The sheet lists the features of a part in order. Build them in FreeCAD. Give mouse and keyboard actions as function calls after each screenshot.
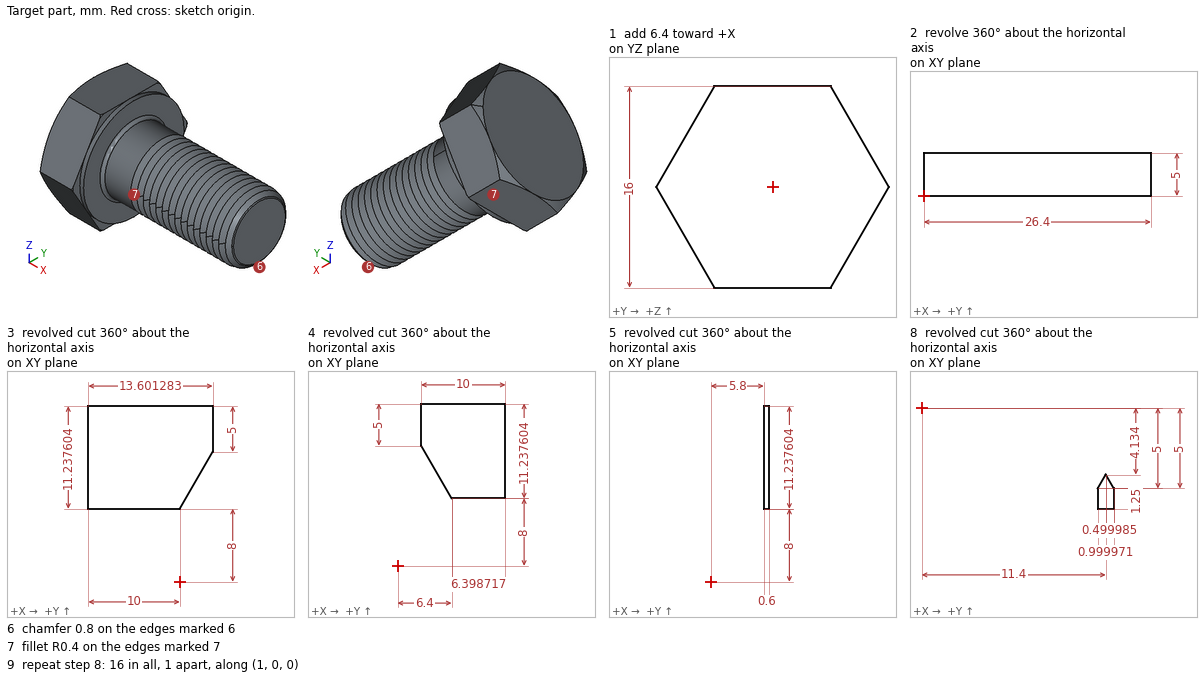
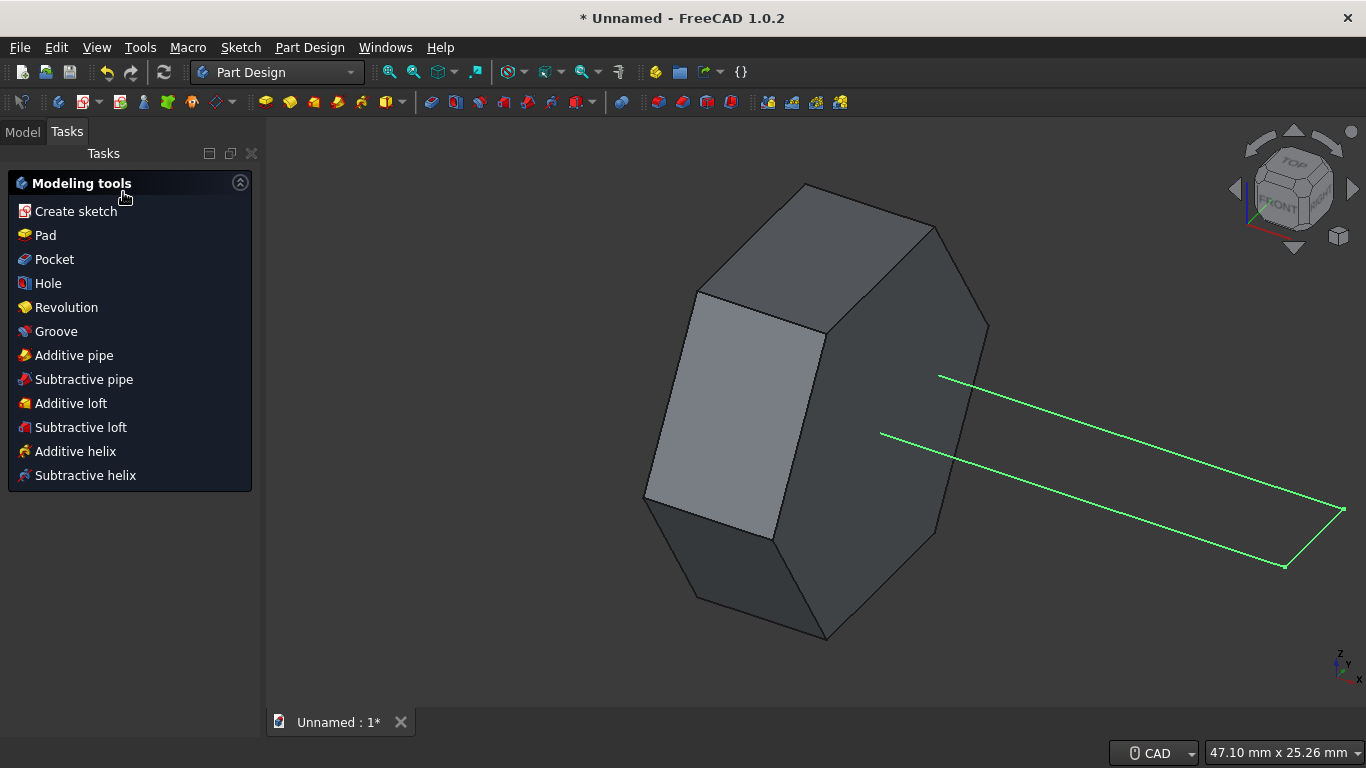
click(290, 102)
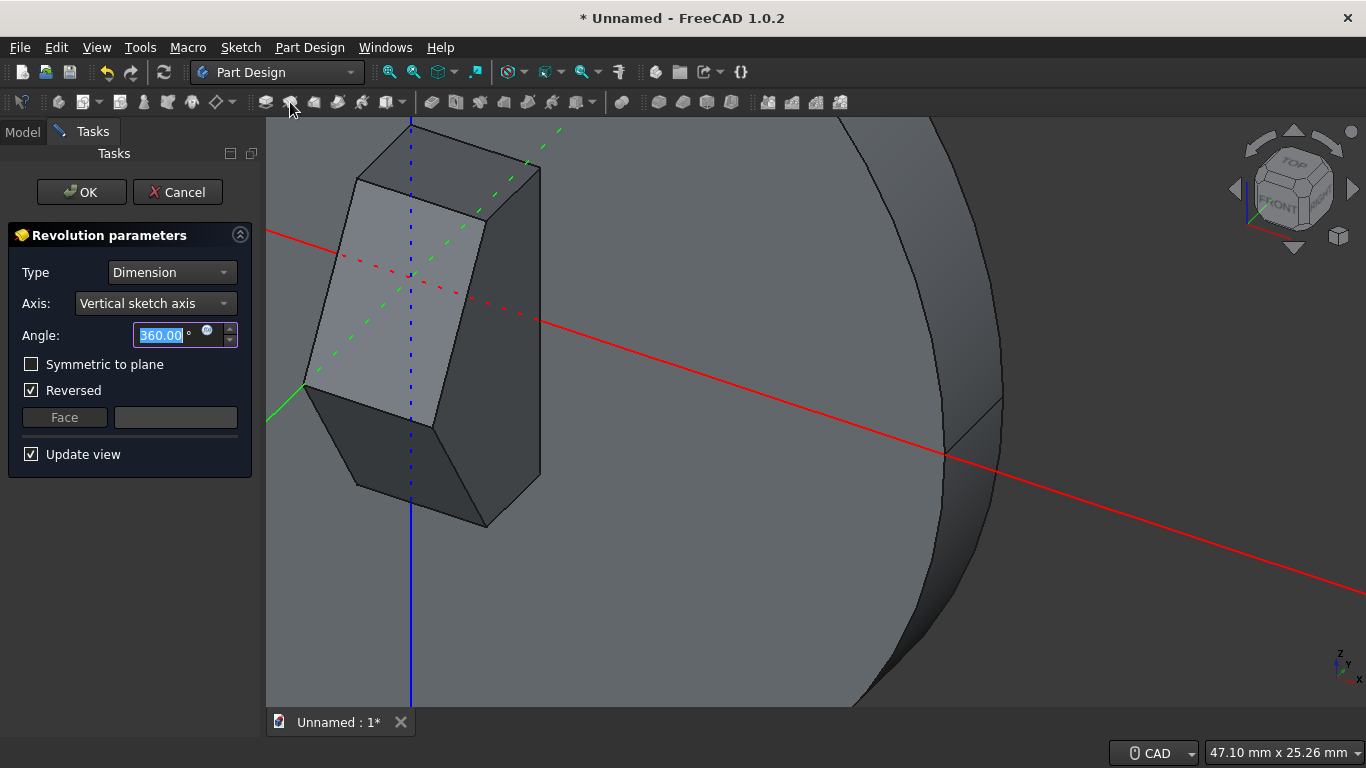
click(156, 304)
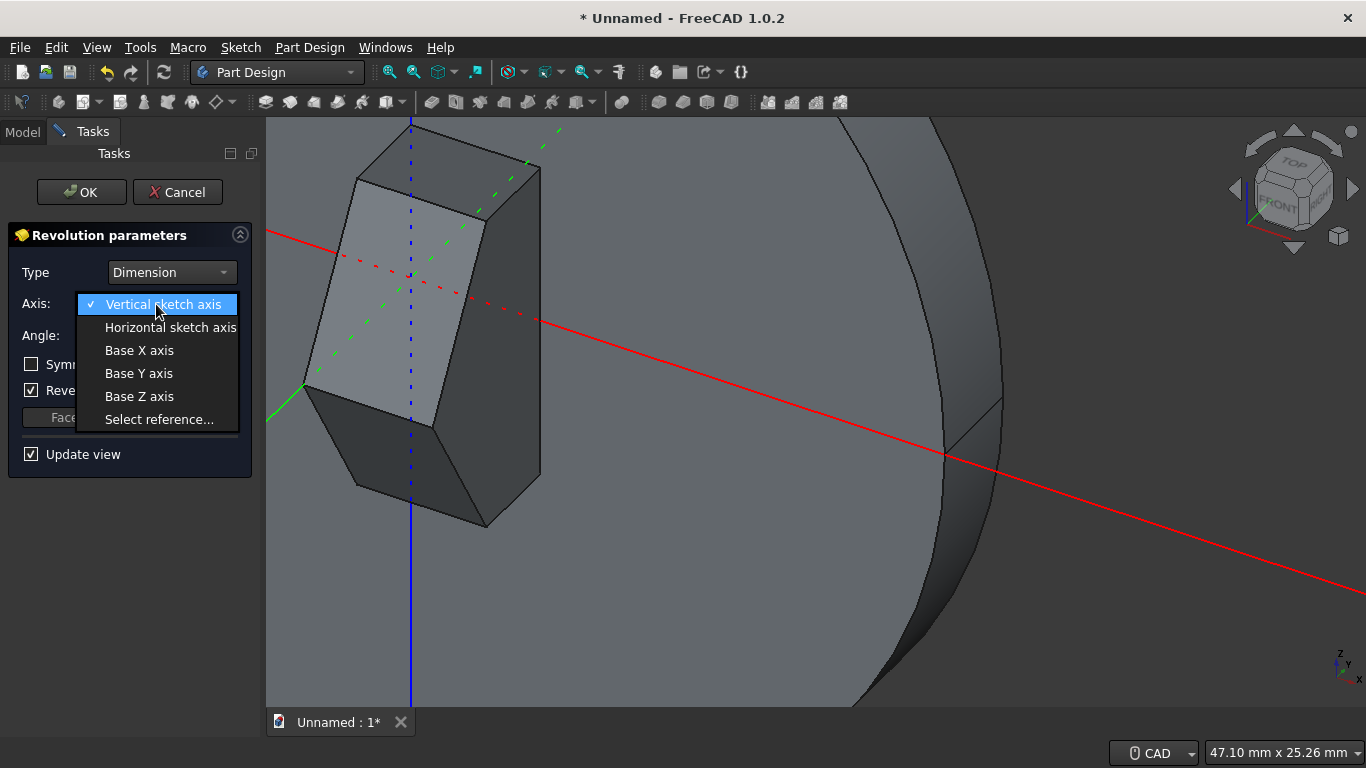
click(156, 328)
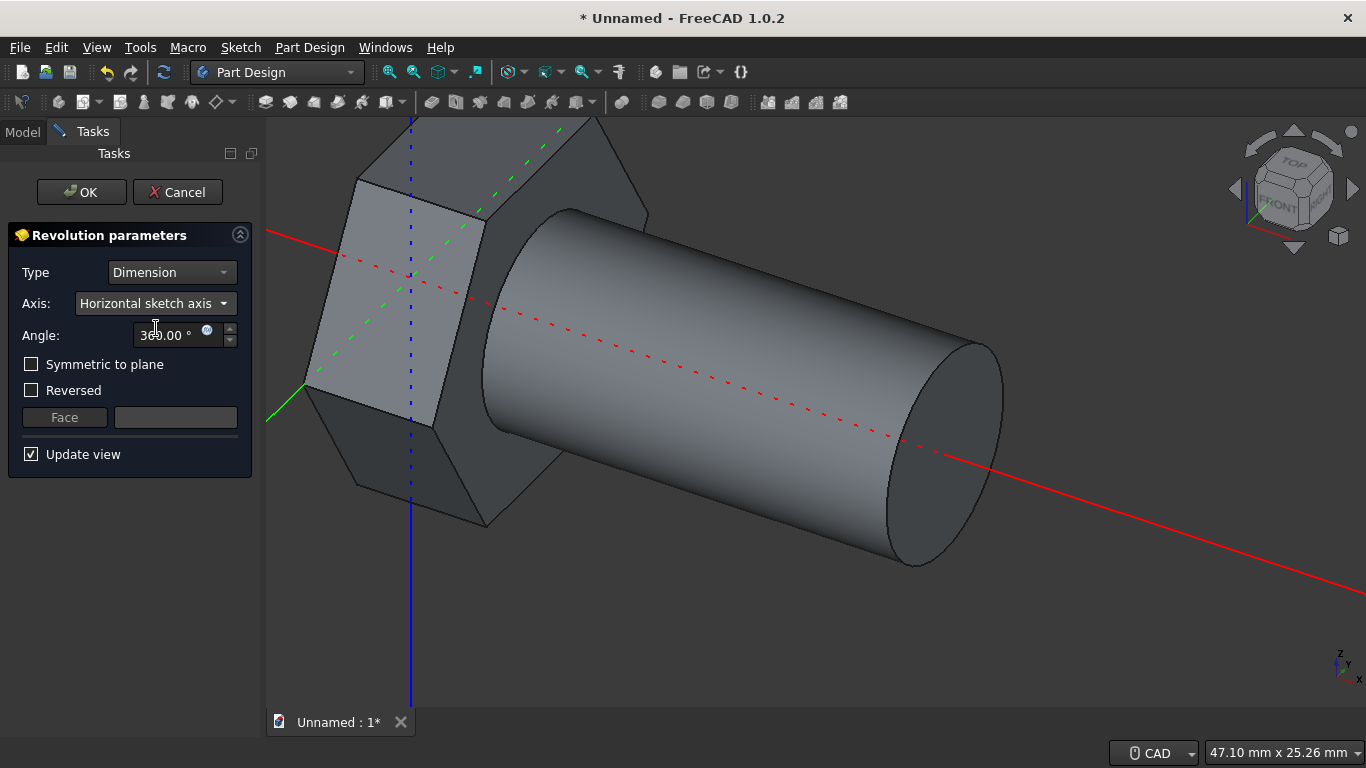
click(82, 192)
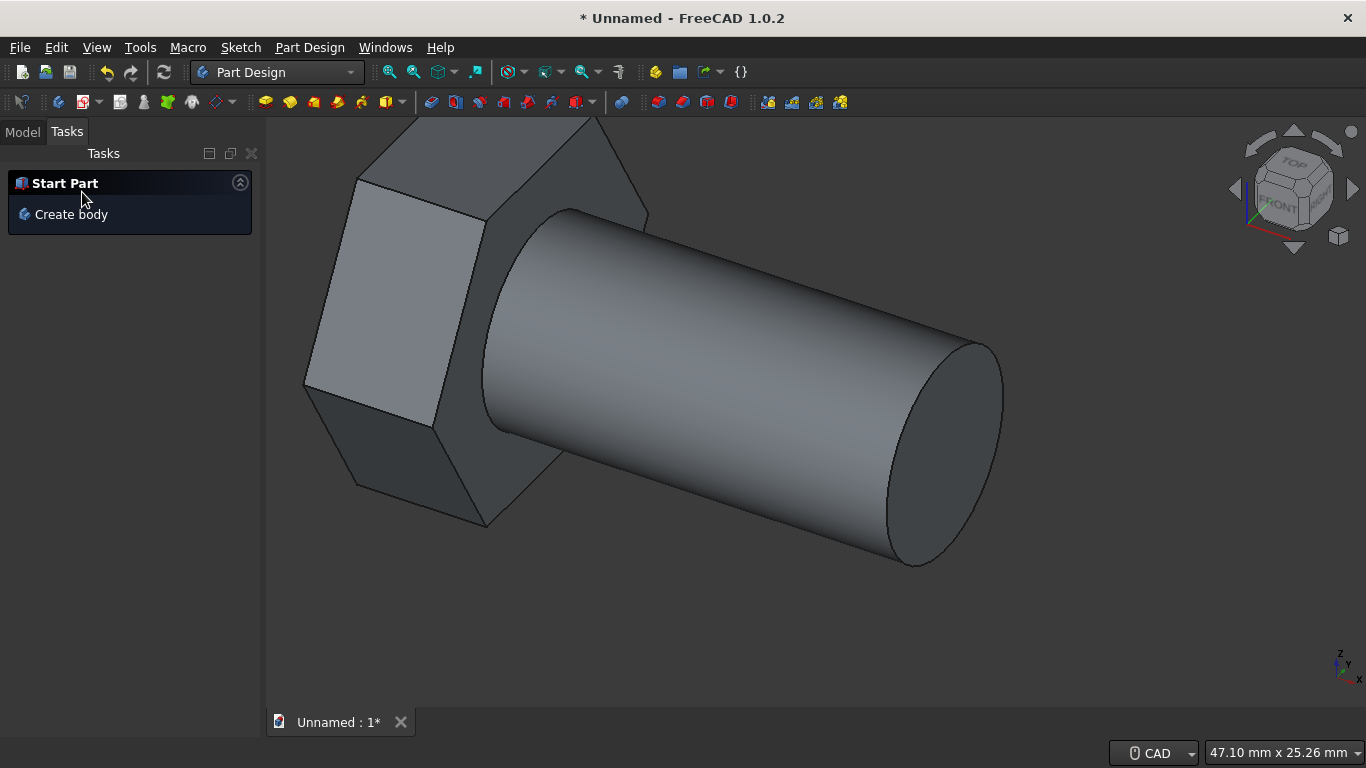
key(v)
key(f)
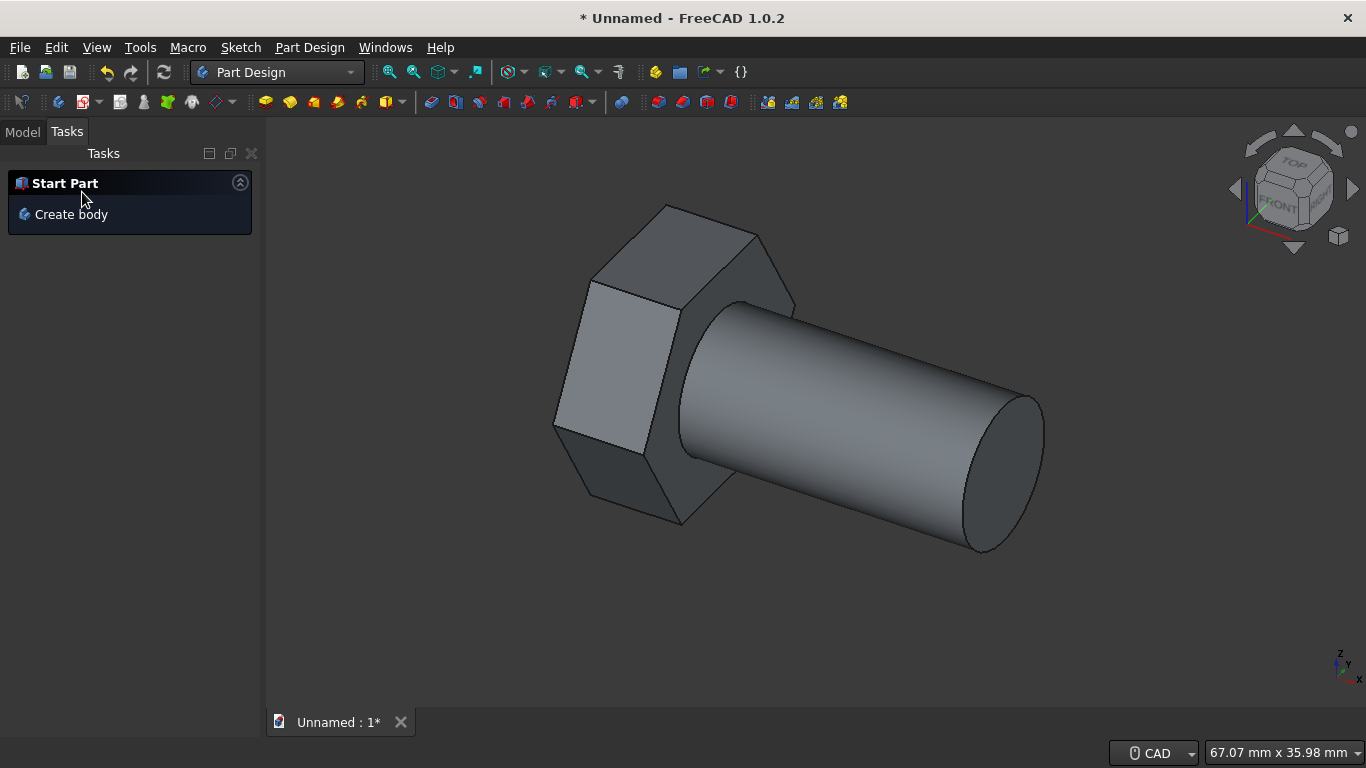
click(84, 102)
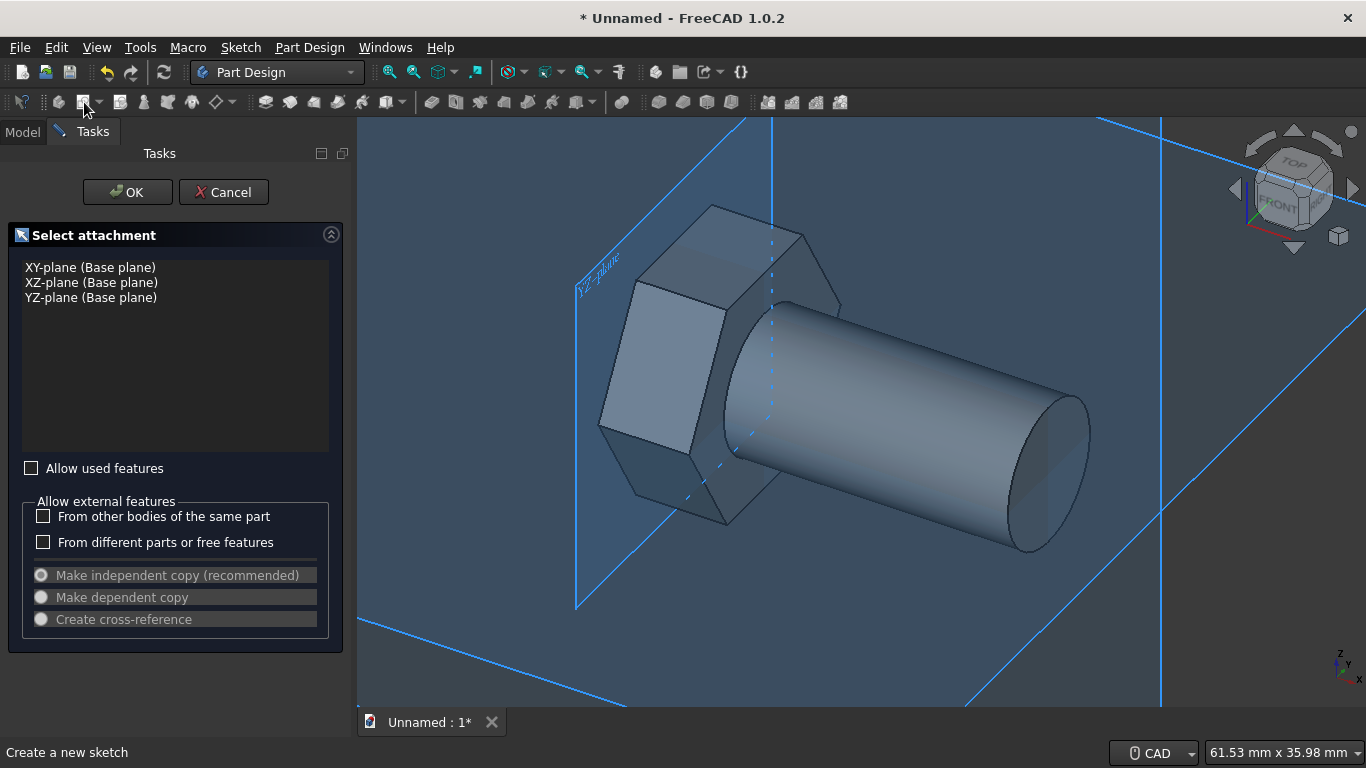
click(82, 268)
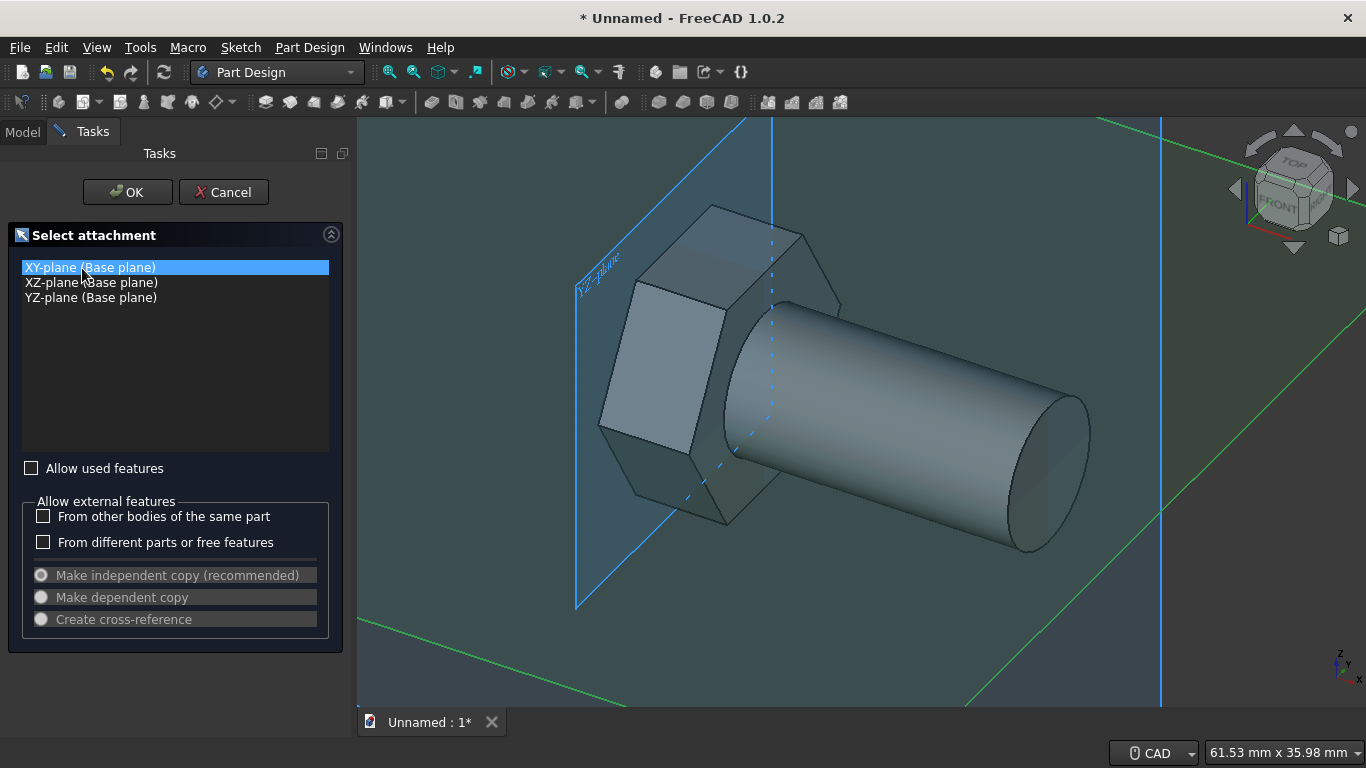
click(128, 192)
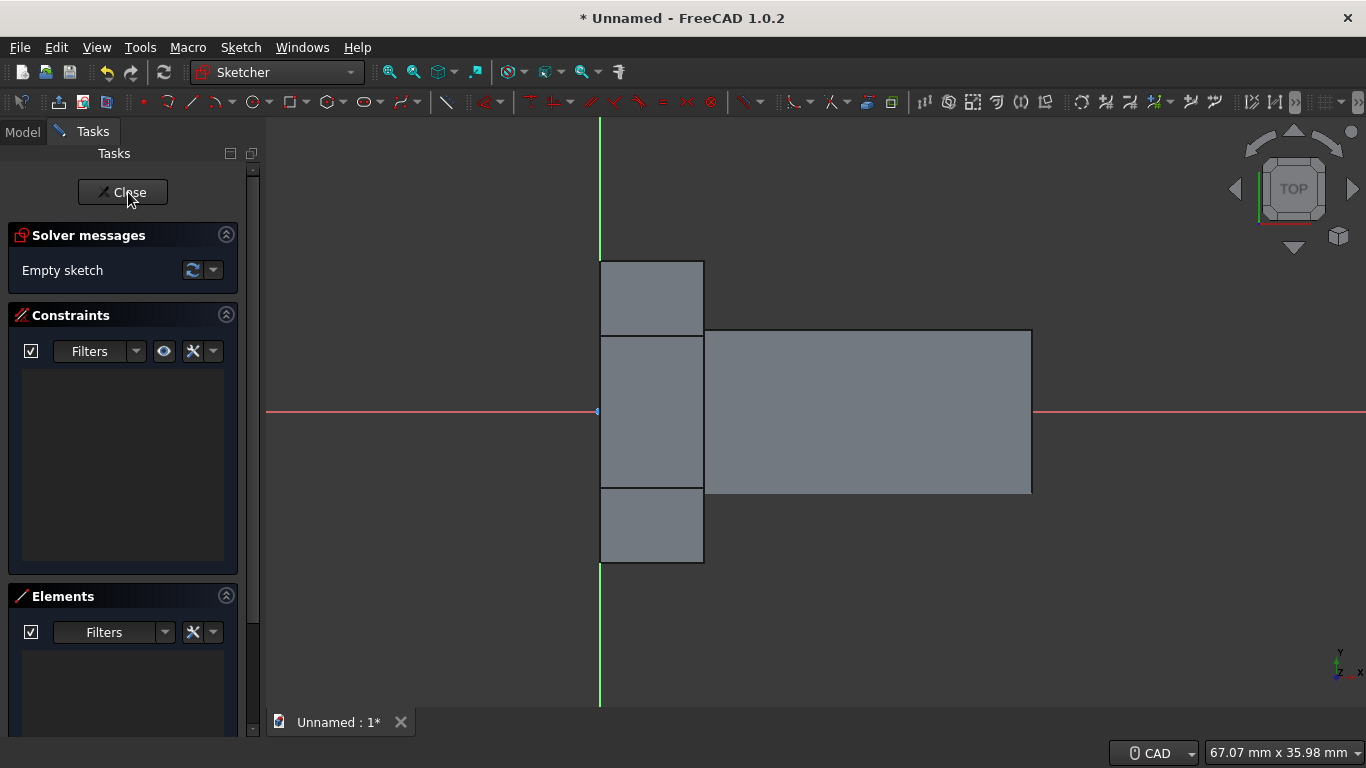
key(q)
key(s)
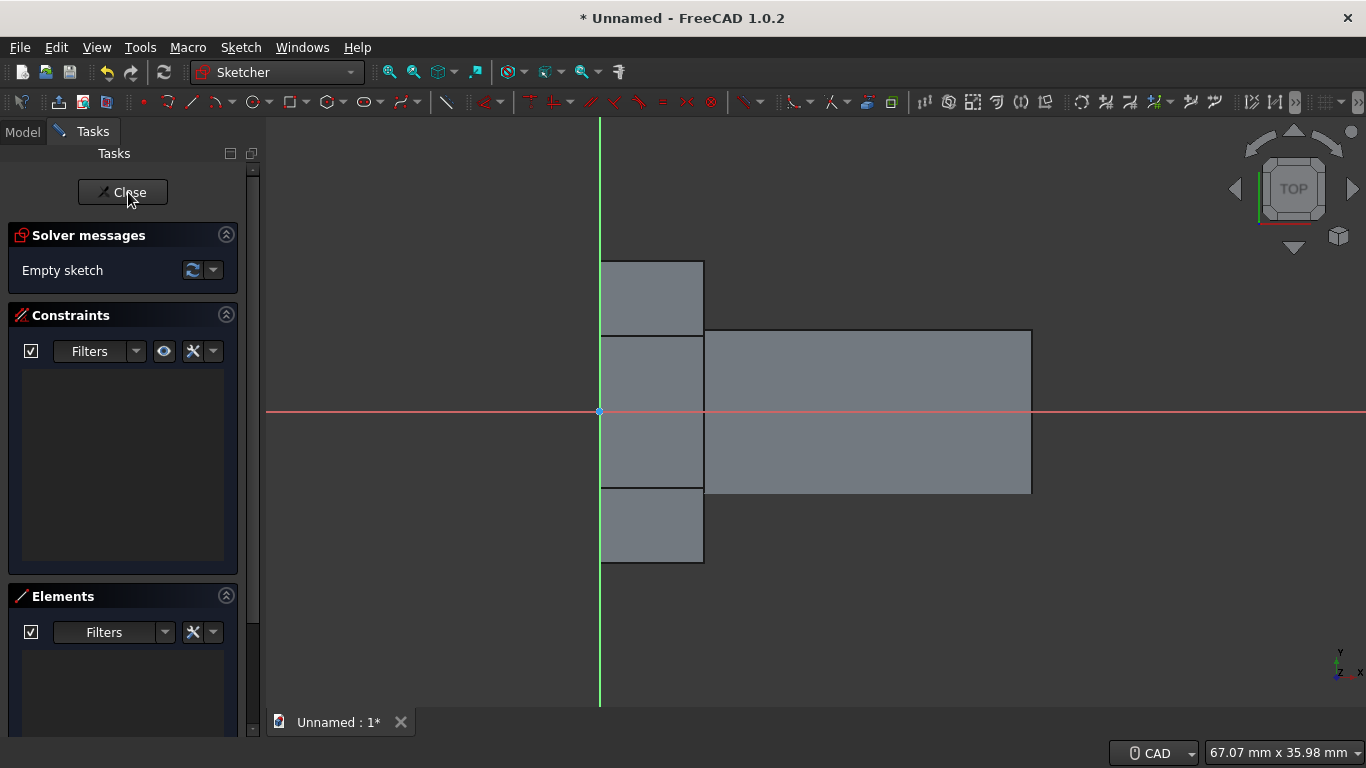
scroll(1201, 679, down, 1)